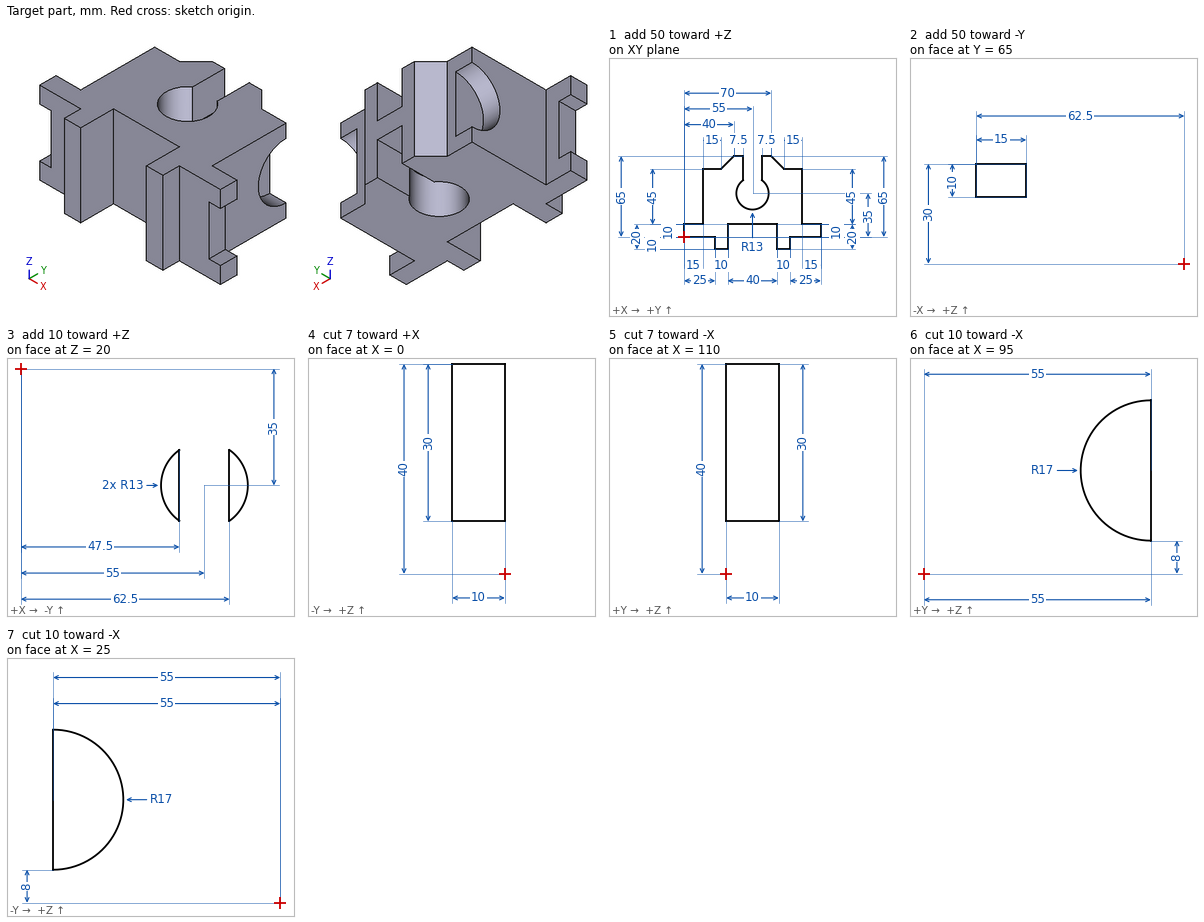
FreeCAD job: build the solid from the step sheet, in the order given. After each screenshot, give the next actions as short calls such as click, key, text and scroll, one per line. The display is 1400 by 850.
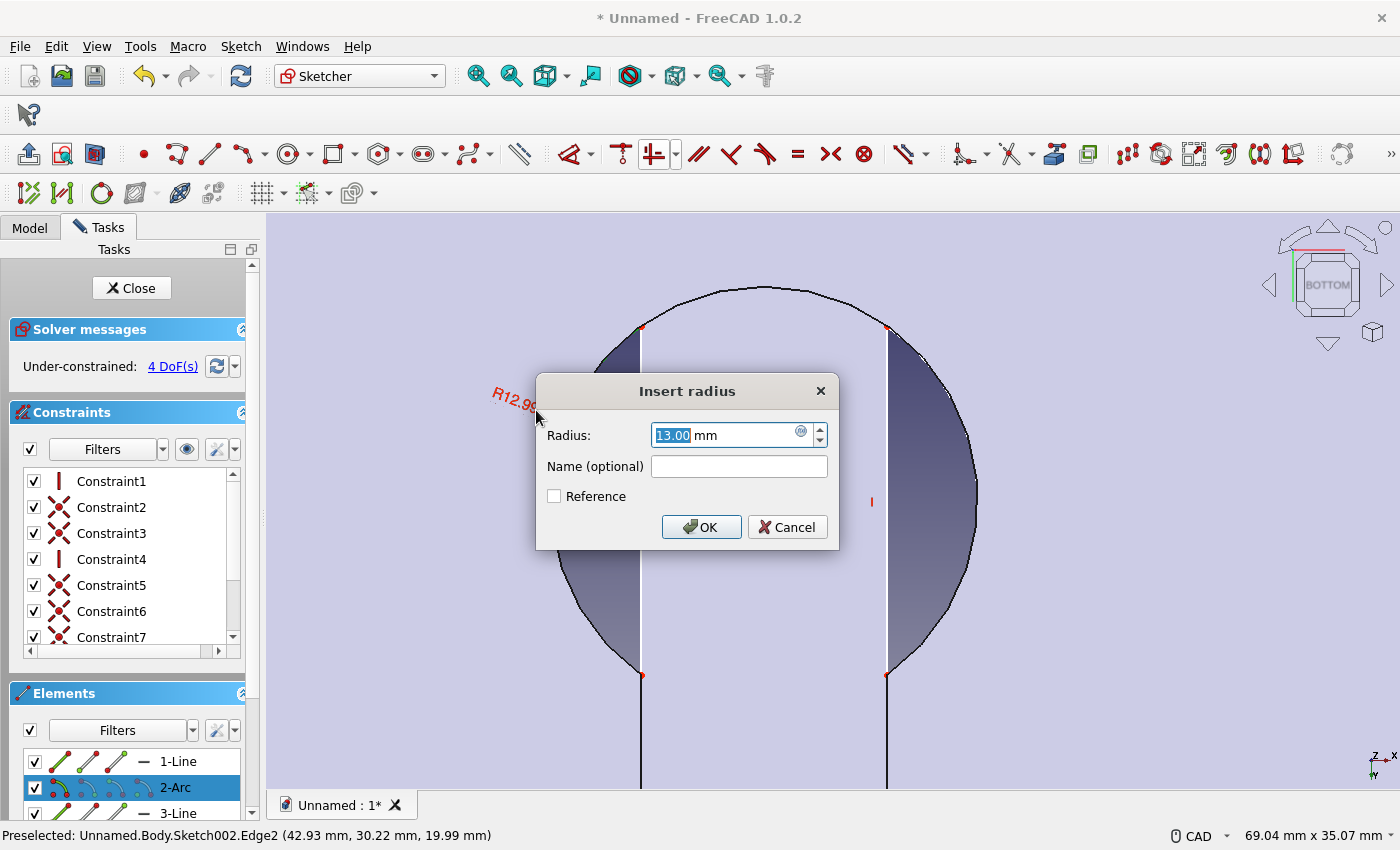
text(13)
key(Return)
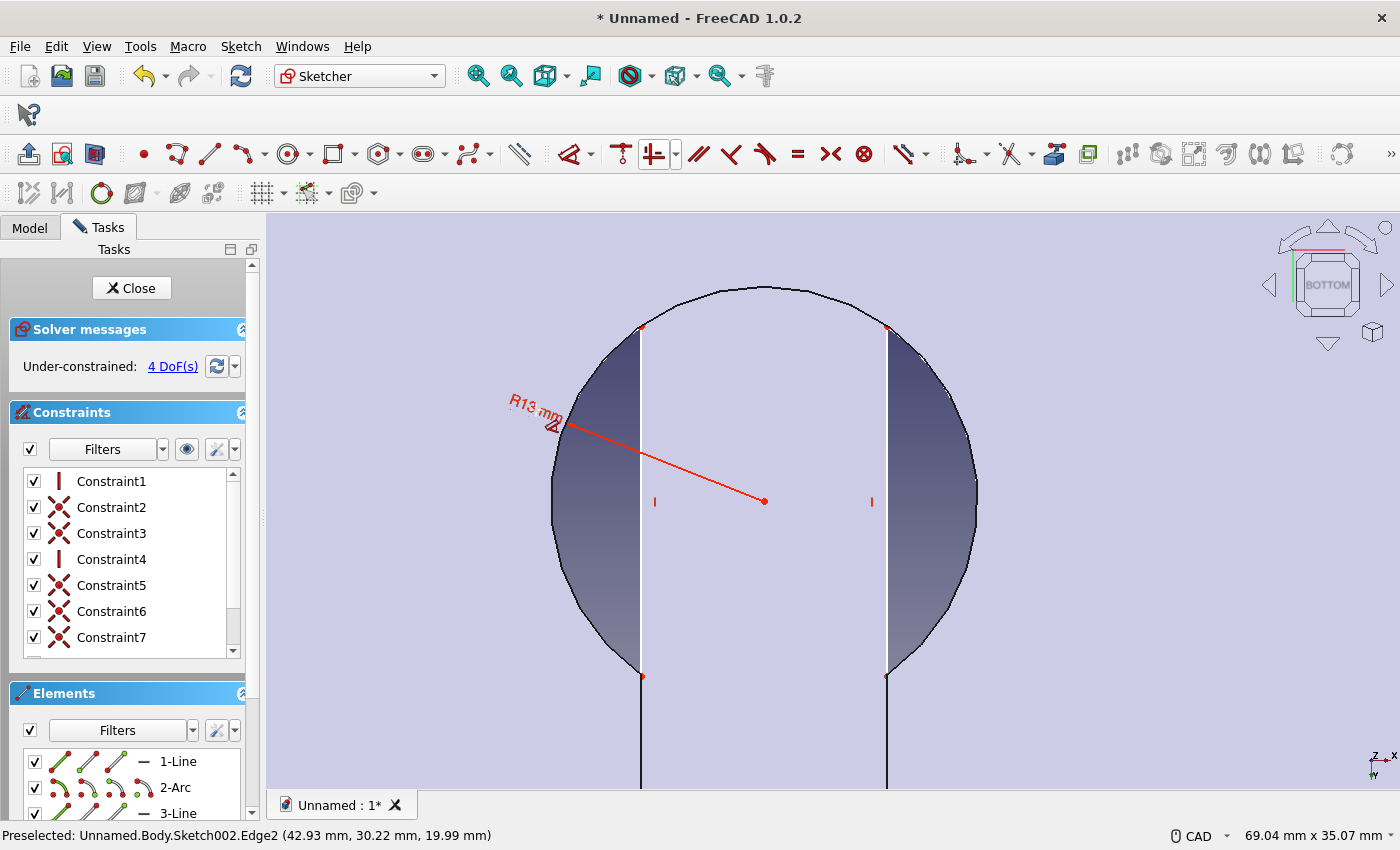
click(764, 502)
click(529, 536)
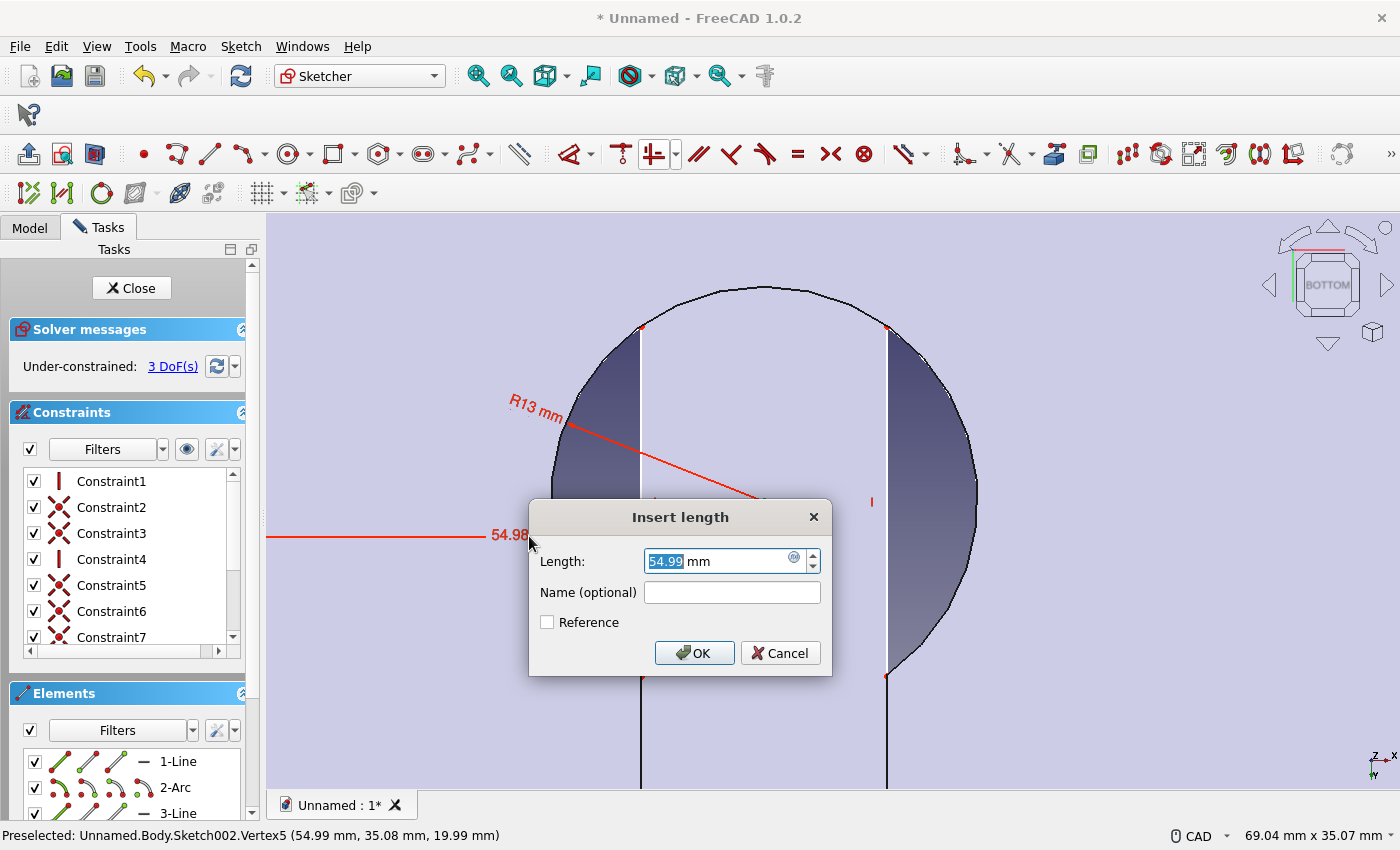
text(55)
key(Return)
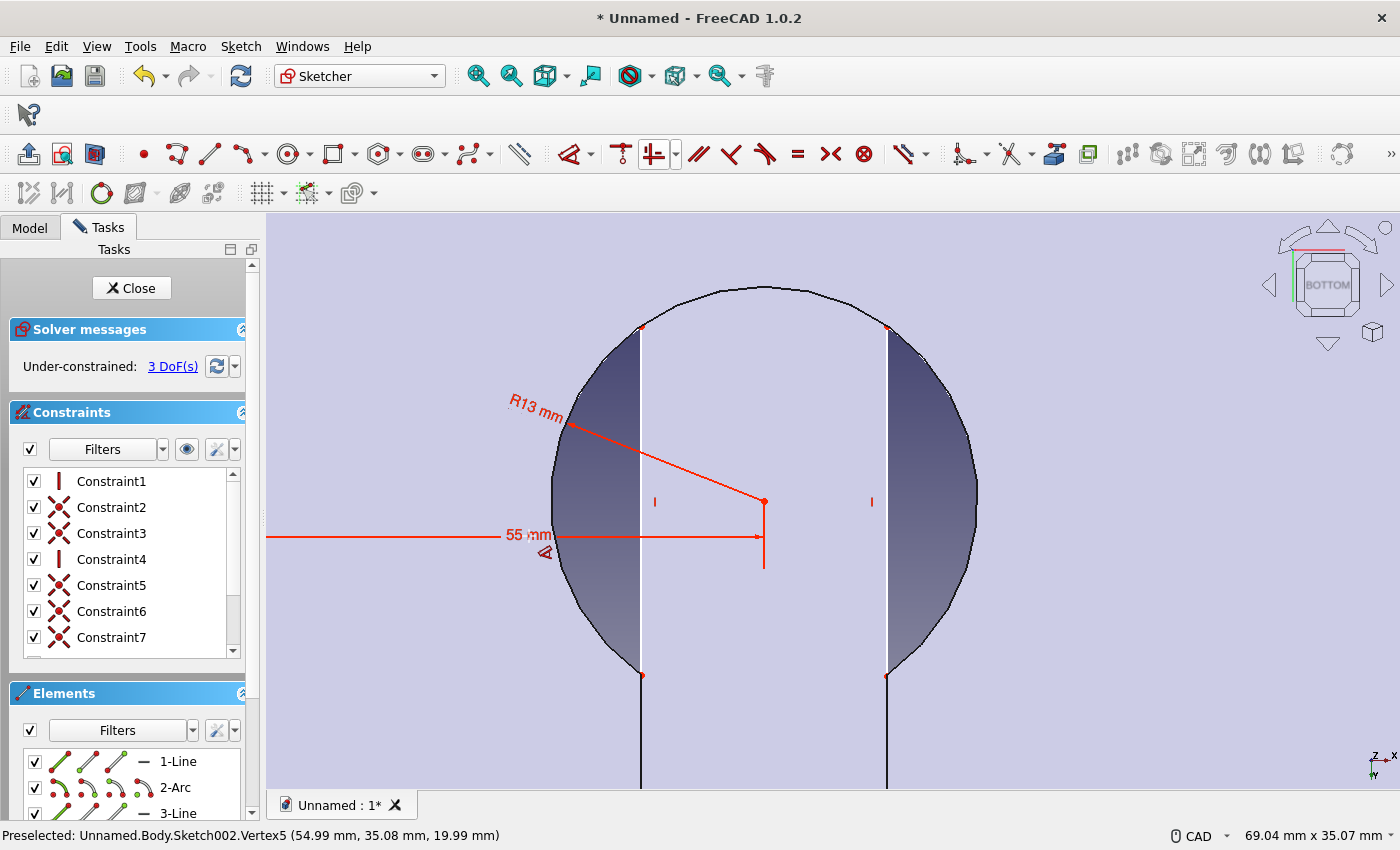
click(764, 501)
click(798, 371)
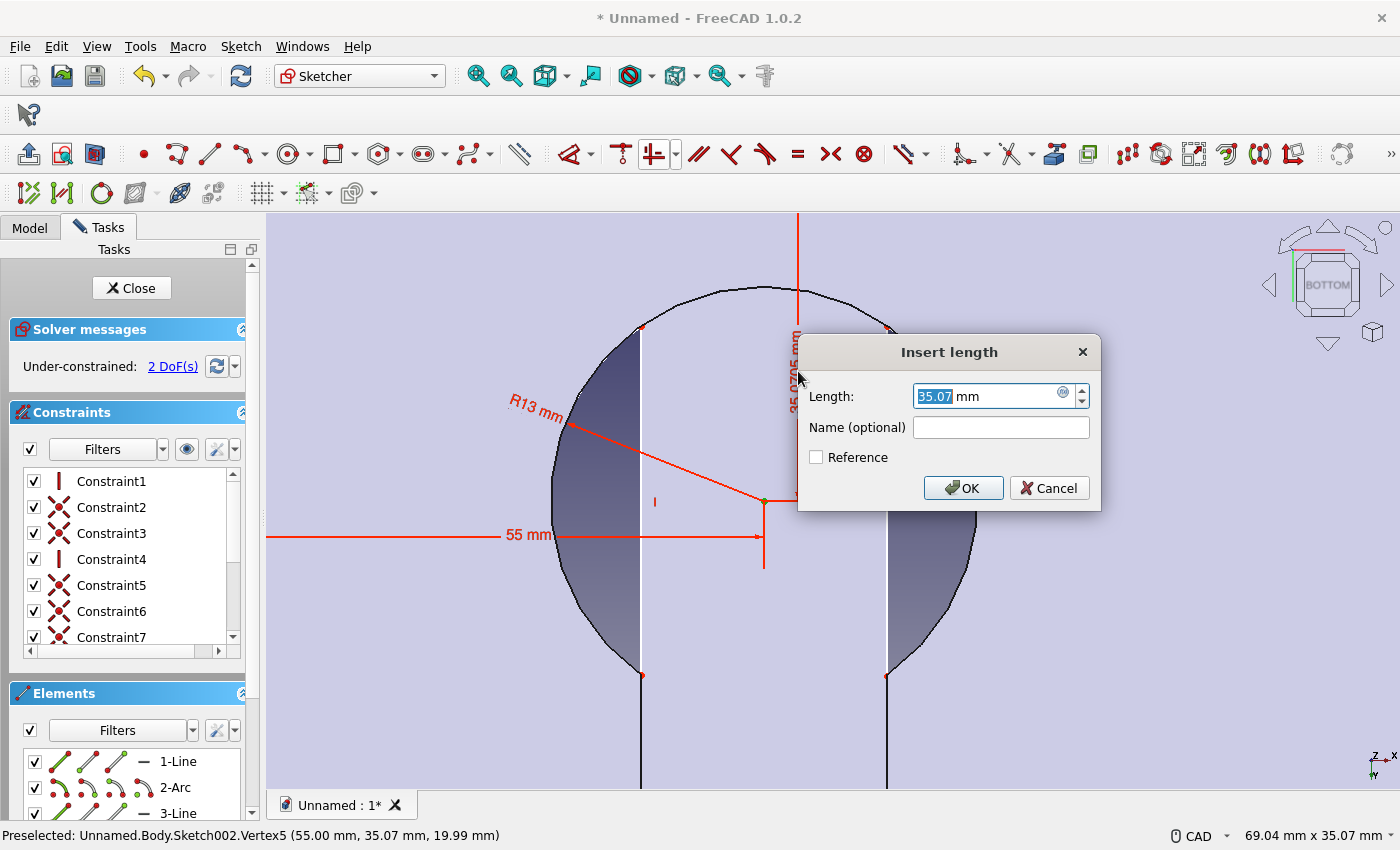
text(35)
key(Return)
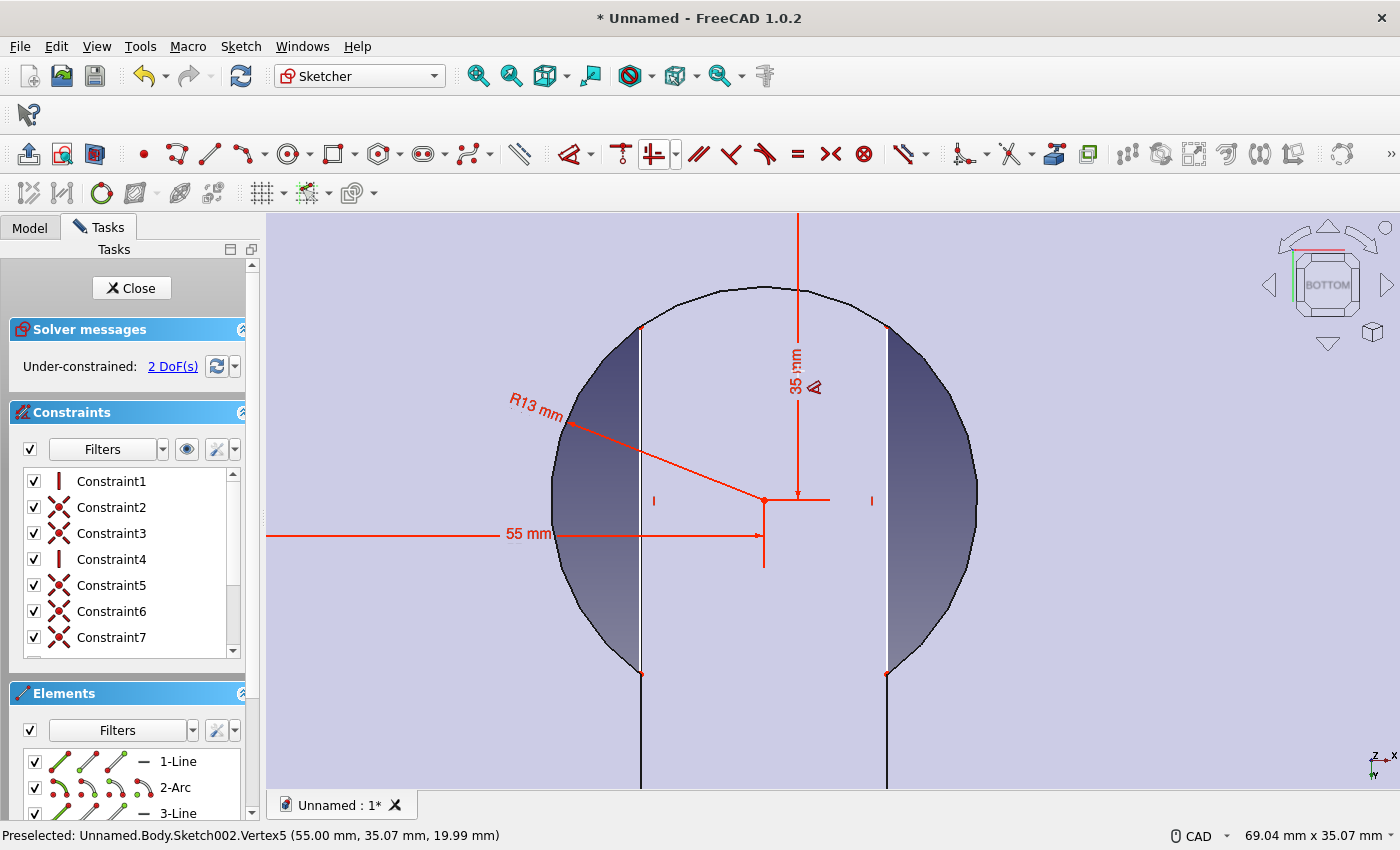
click(640, 326)
click(467, 360)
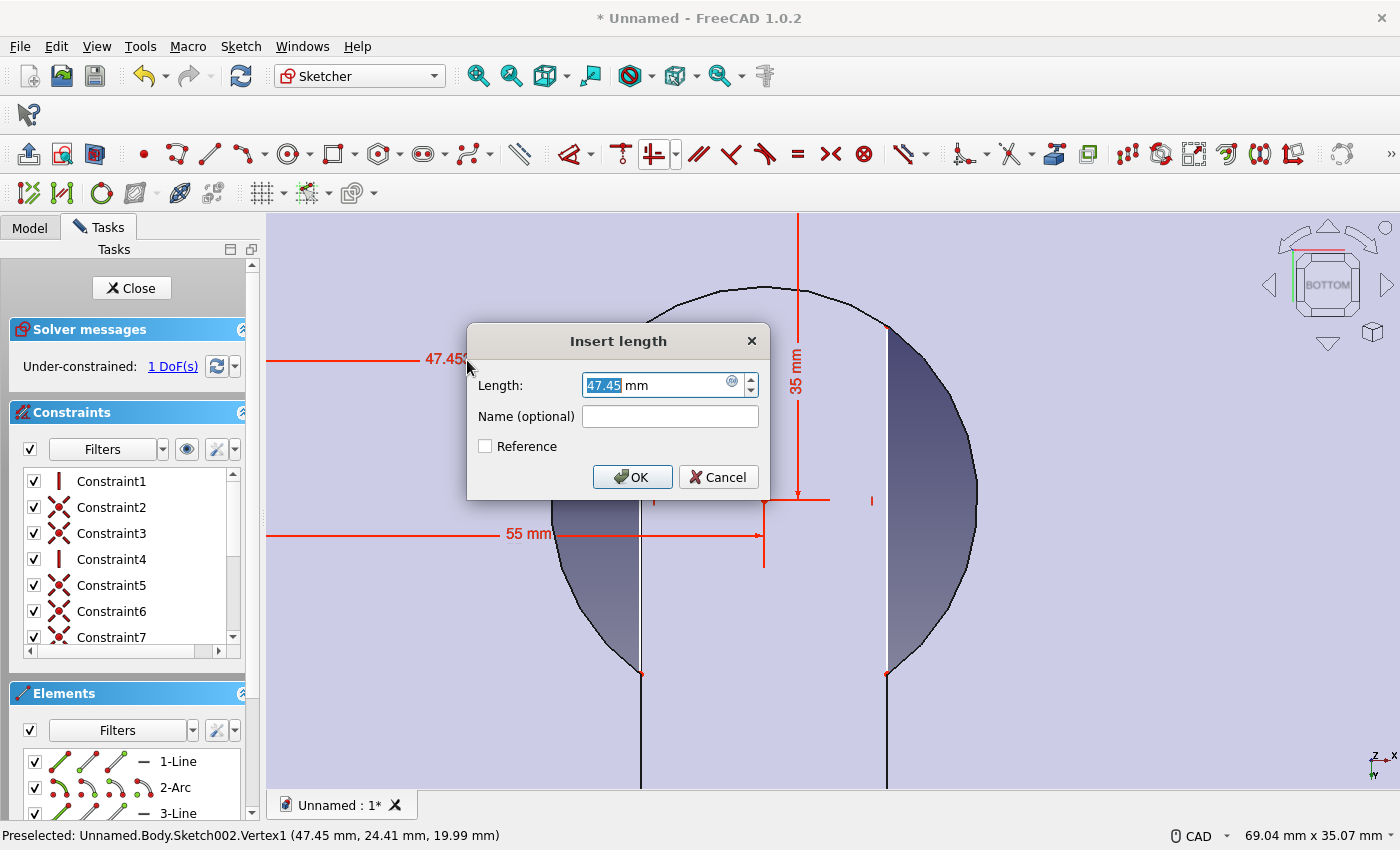
text(47.5)
key(Return)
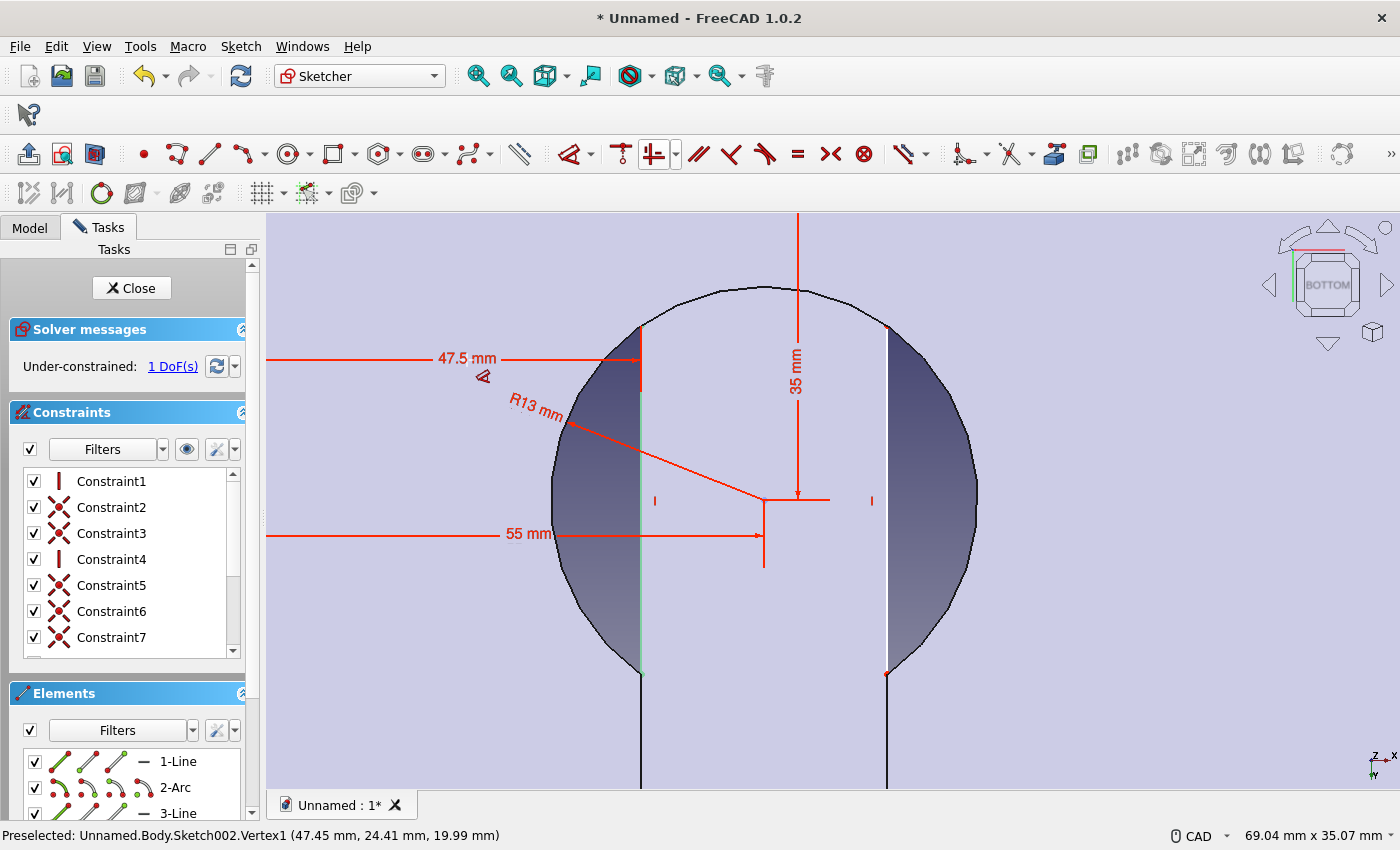
click(887, 675)
click(590, 709)